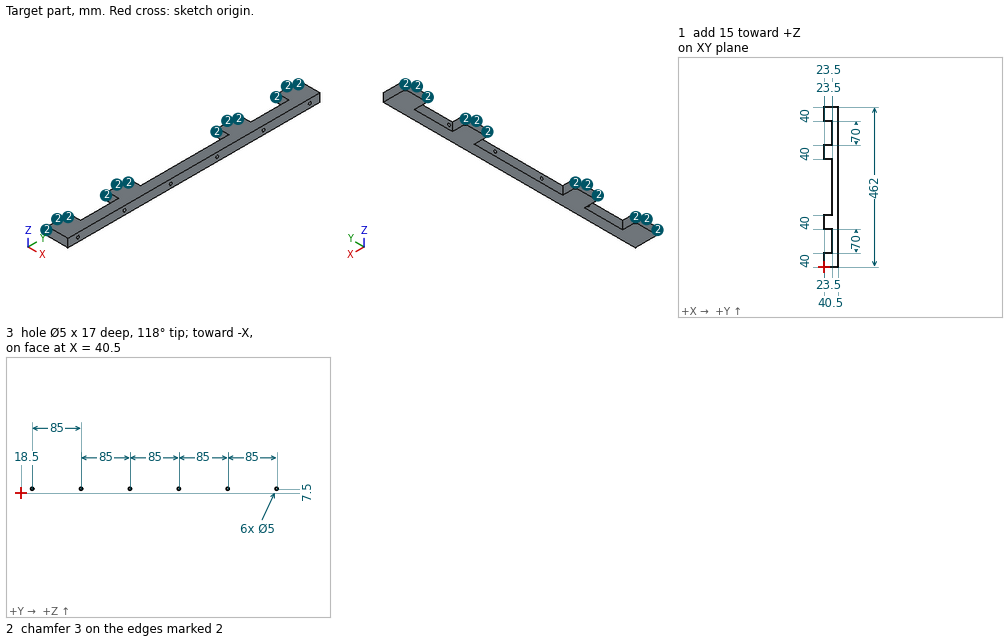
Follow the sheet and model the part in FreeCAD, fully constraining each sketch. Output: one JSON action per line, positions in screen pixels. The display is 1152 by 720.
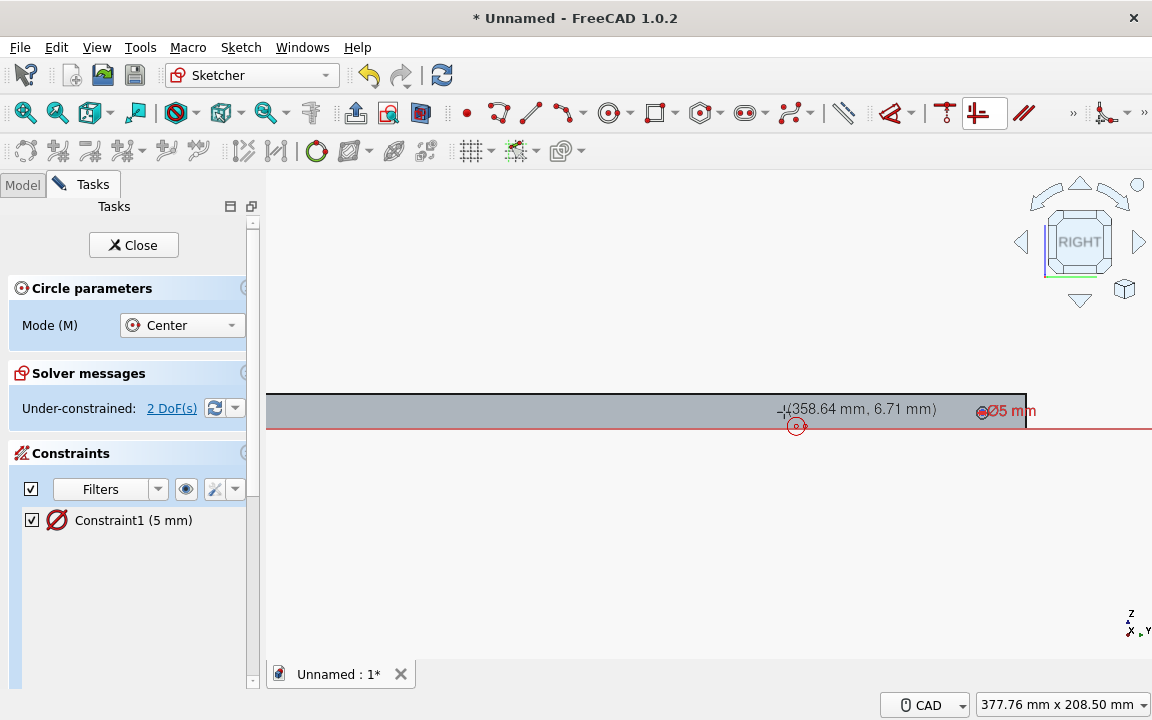
{"action": "left_click", "coordinate": [783, 412]}
{"action": "mouse_move", "coordinate": [787, 408]}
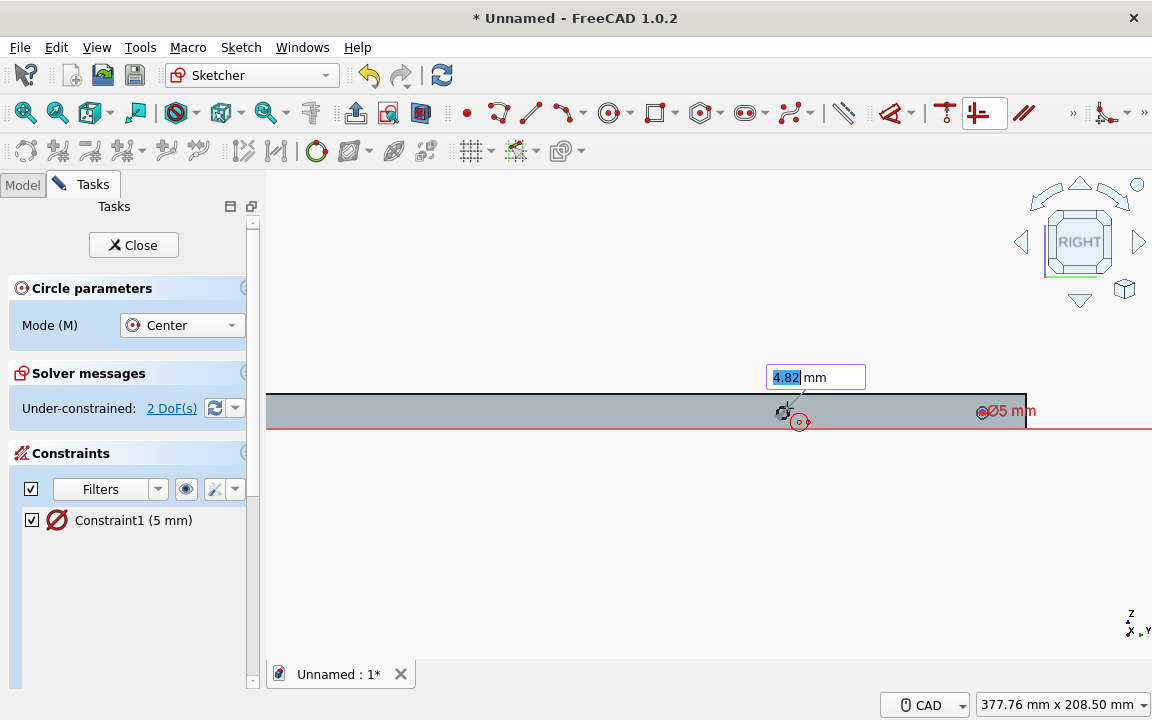
{"action": "type", "text": "5"}
{"action": "key", "text": "Return"}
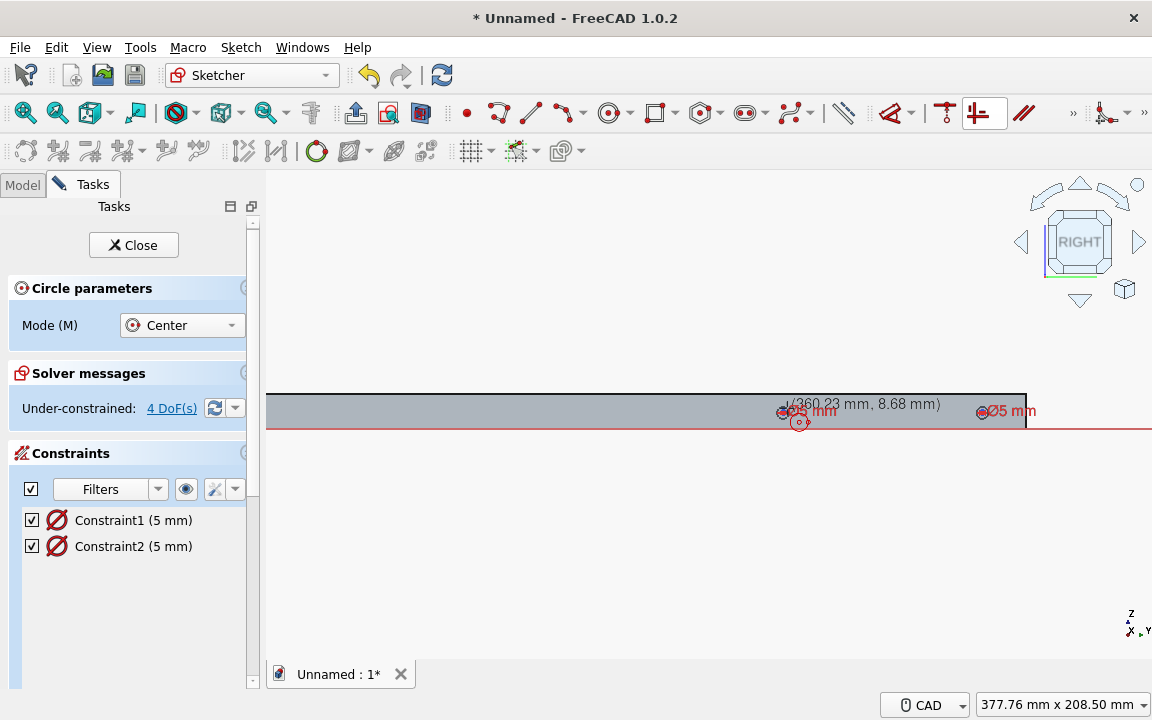
{"action": "scroll", "coordinate": [584, 412], "scroll_direction": "up", "scroll_amount": 7}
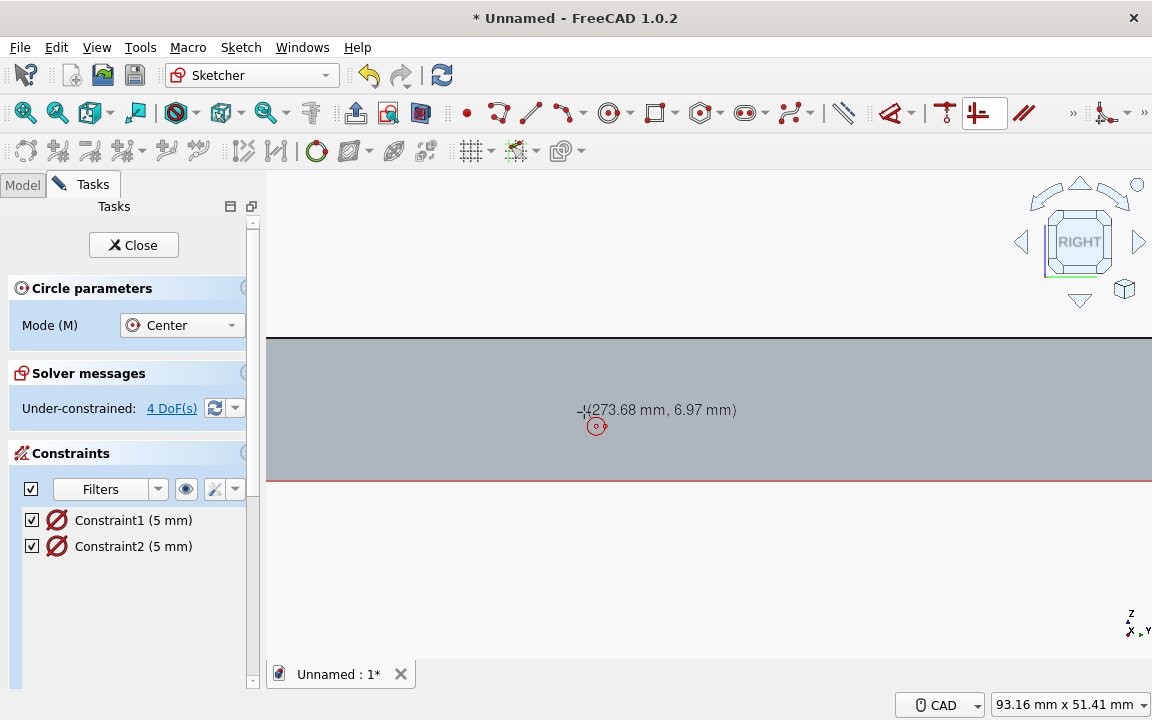
{"action": "scroll", "coordinate": [708, 412], "scroll_direction": "down", "scroll_amount": 11}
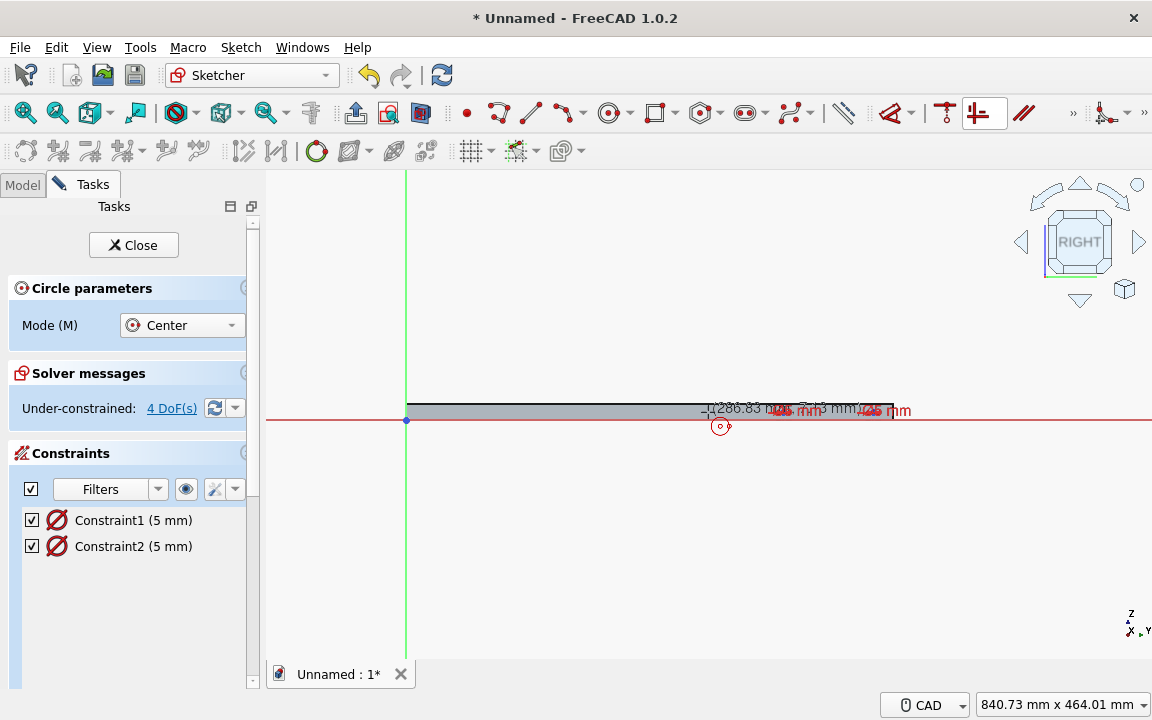
{"action": "scroll", "coordinate": [694, 412], "scroll_direction": "up", "scroll_amount": 4}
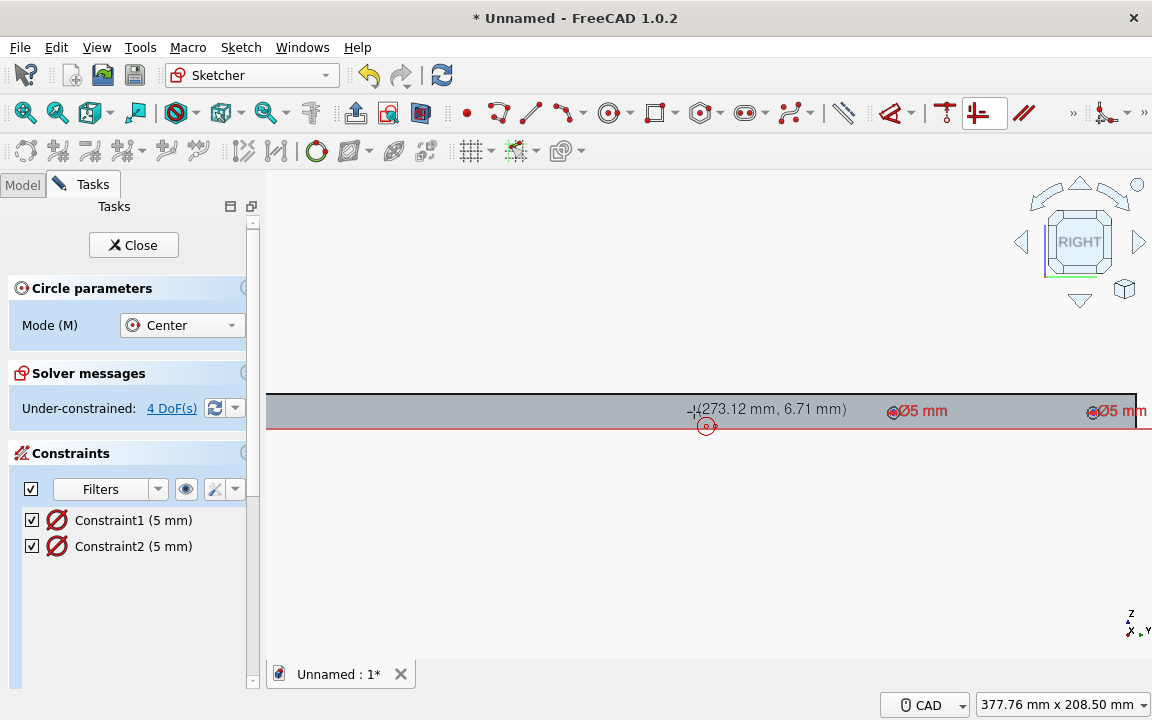
{"action": "left_click", "coordinate": [694, 412]}
{"action": "mouse_move", "coordinate": [698, 408]}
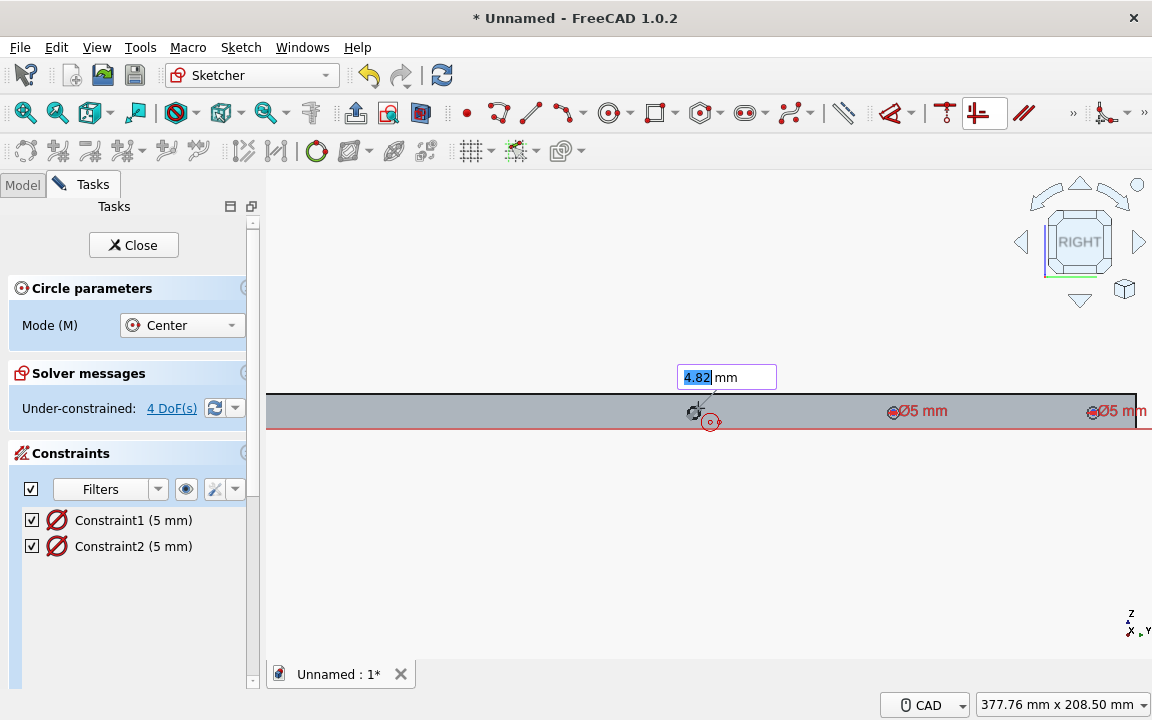
{"action": "type", "text": "5"}
{"action": "key", "text": "Return"}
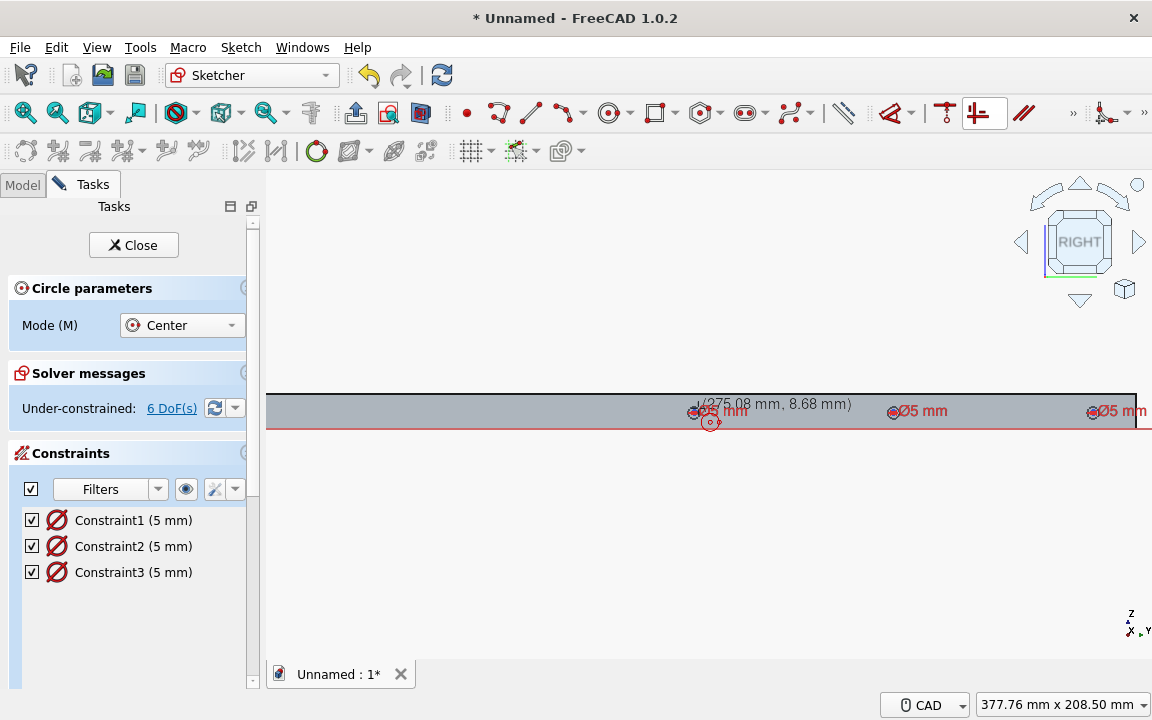
{"action": "scroll", "coordinate": [495, 412], "scroll_direction": "up", "scroll_amount": 7}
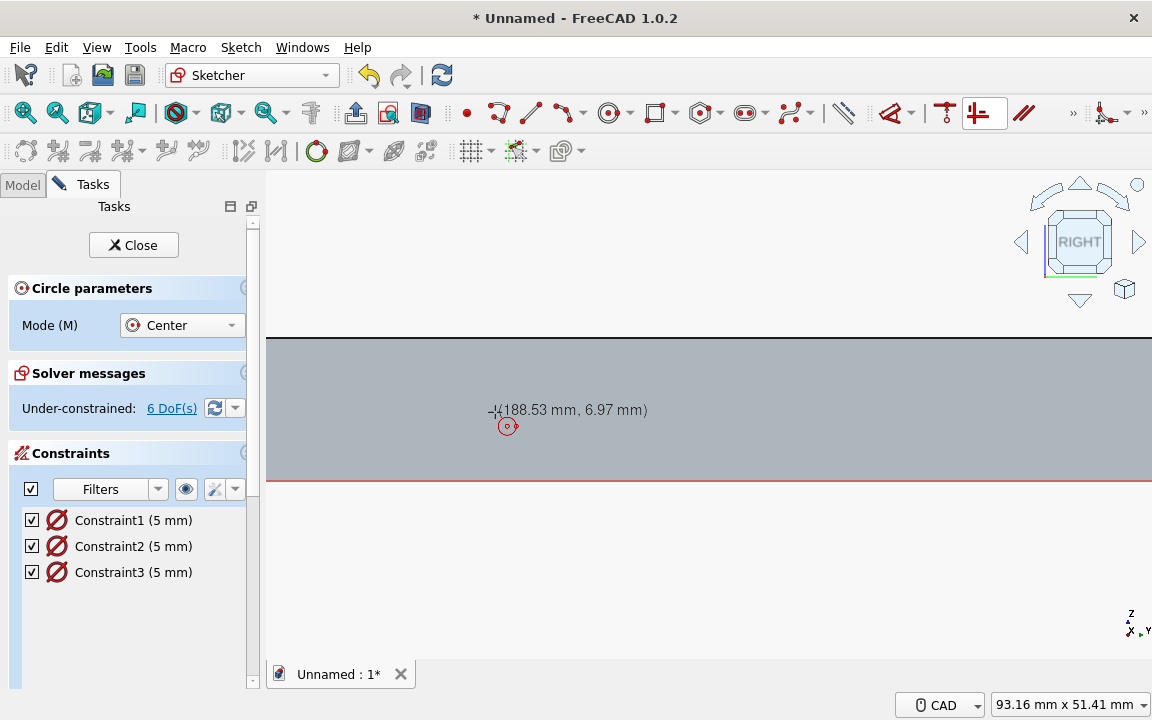
{"action": "scroll", "coordinate": [618, 412], "scroll_direction": "down", "scroll_amount": 11}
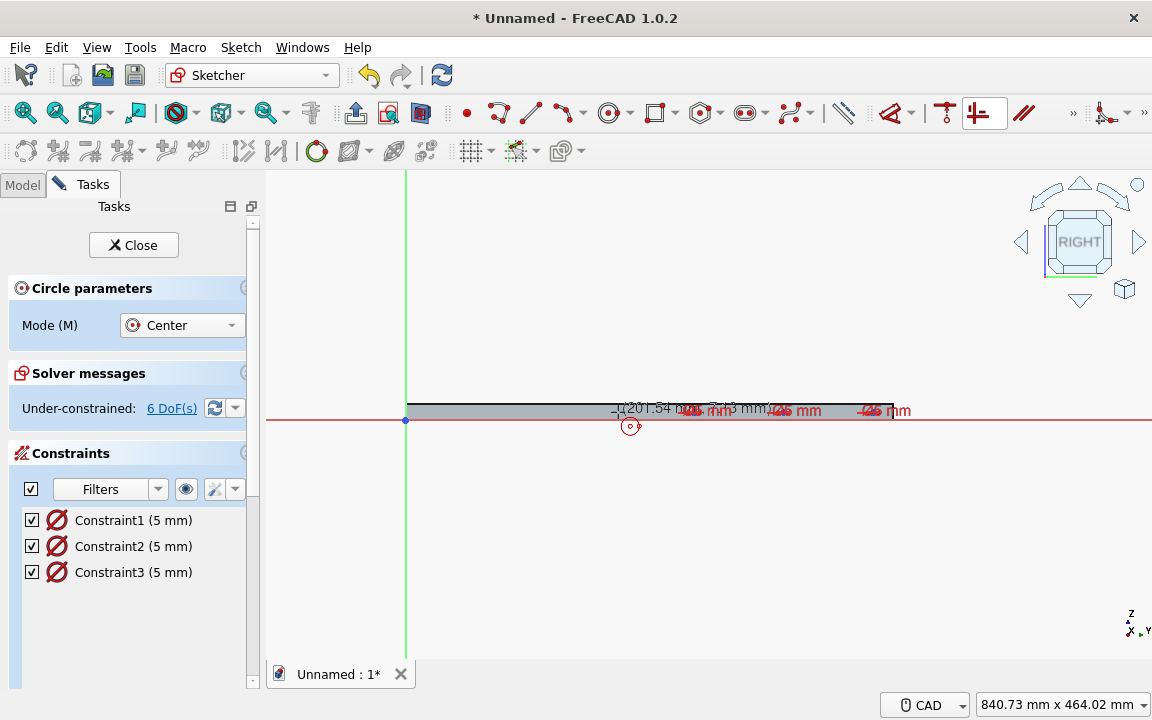
{"action": "scroll", "coordinate": [605, 412], "scroll_direction": "up", "scroll_amount": 4}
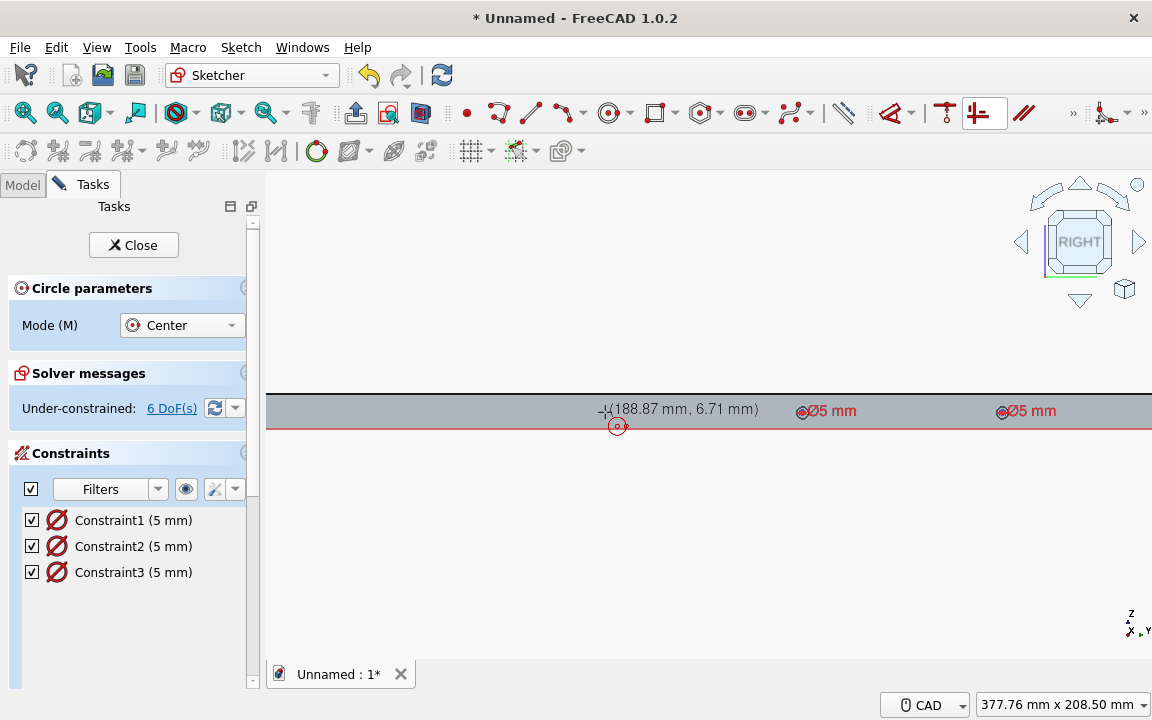
{"action": "left_click", "coordinate": [604, 412]}
{"action": "mouse_move", "coordinate": [608, 408]}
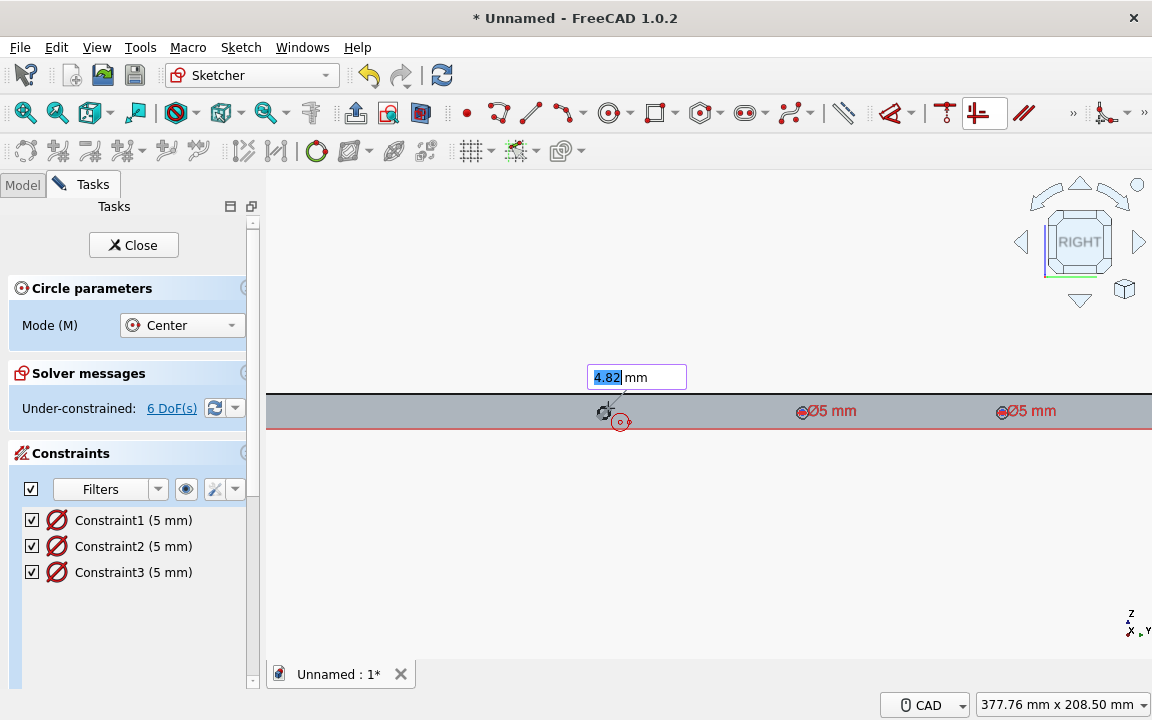
{"action": "type", "text": "5"}
{"action": "key", "text": "Return"}